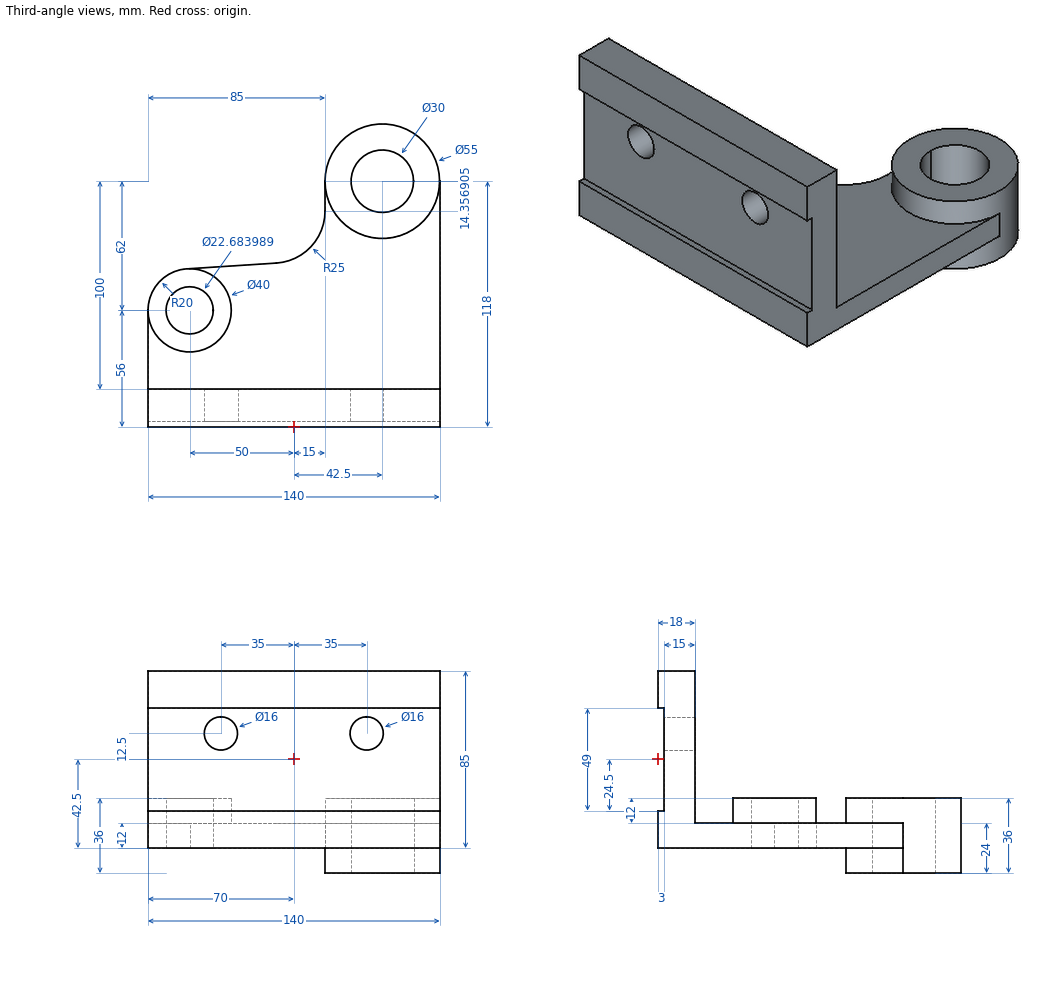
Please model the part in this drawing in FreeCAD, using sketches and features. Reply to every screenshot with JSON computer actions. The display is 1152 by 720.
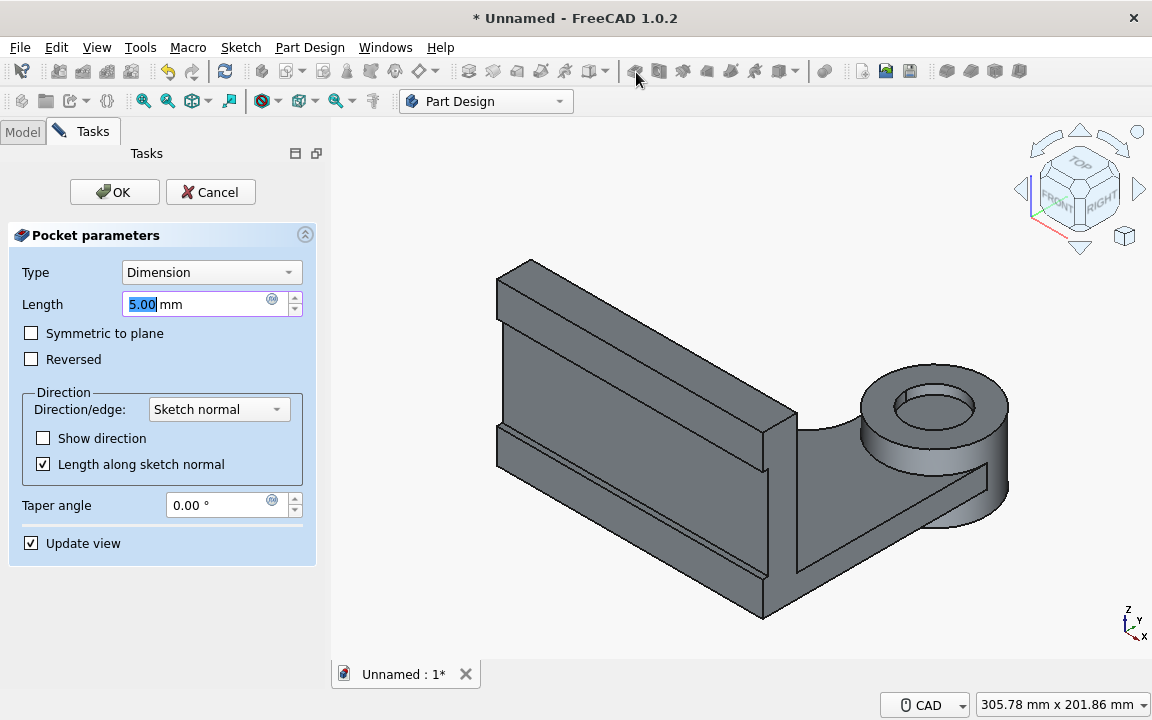
{"action": "type", "text": "36"}
{"action": "key", "text": "Tab"}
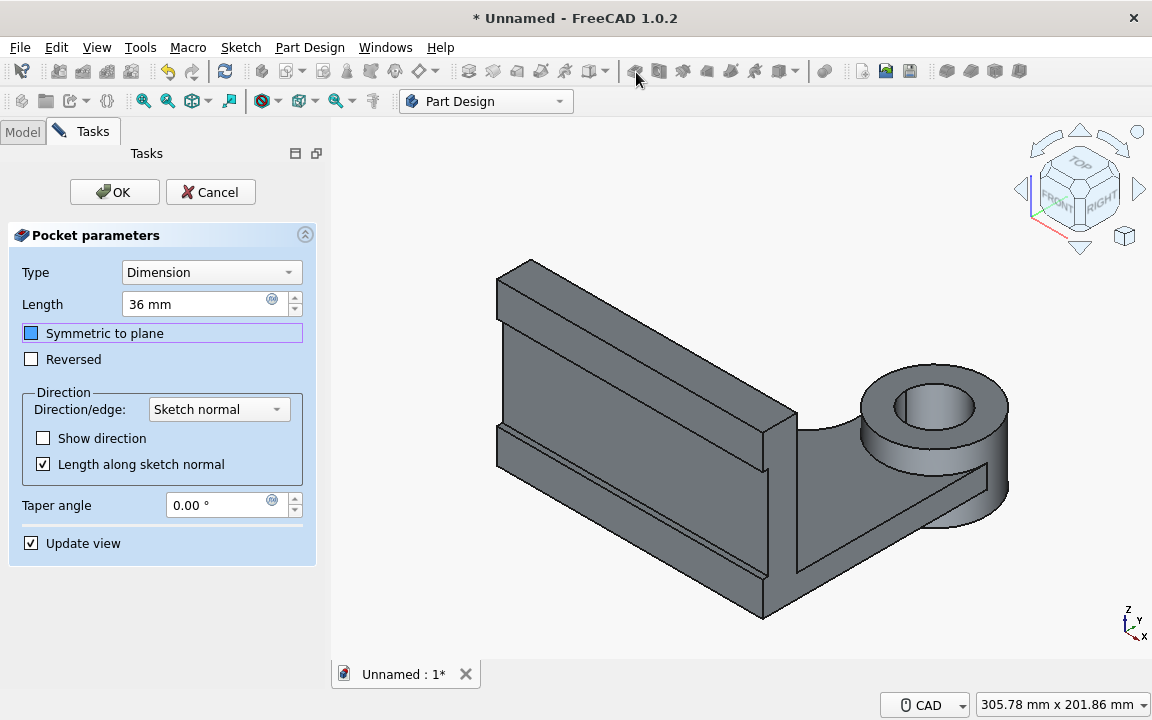
{"action": "left_click", "coordinate": [115, 192]}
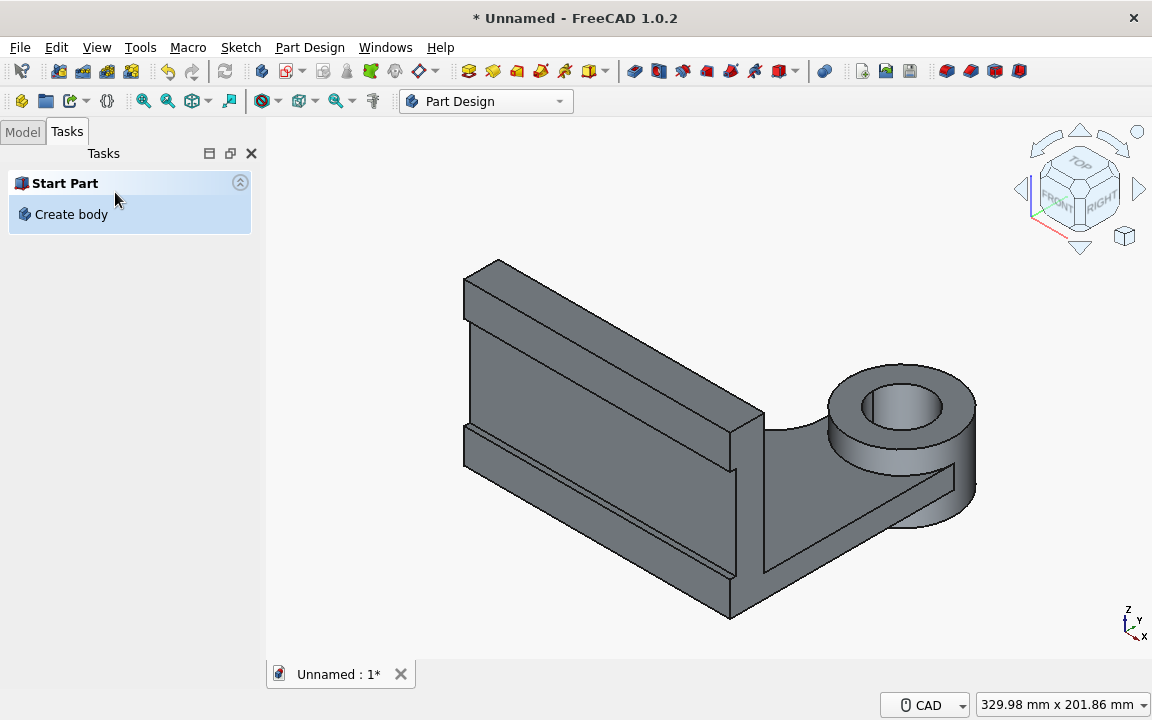
{"action": "left_click", "coordinate": [962, 406]}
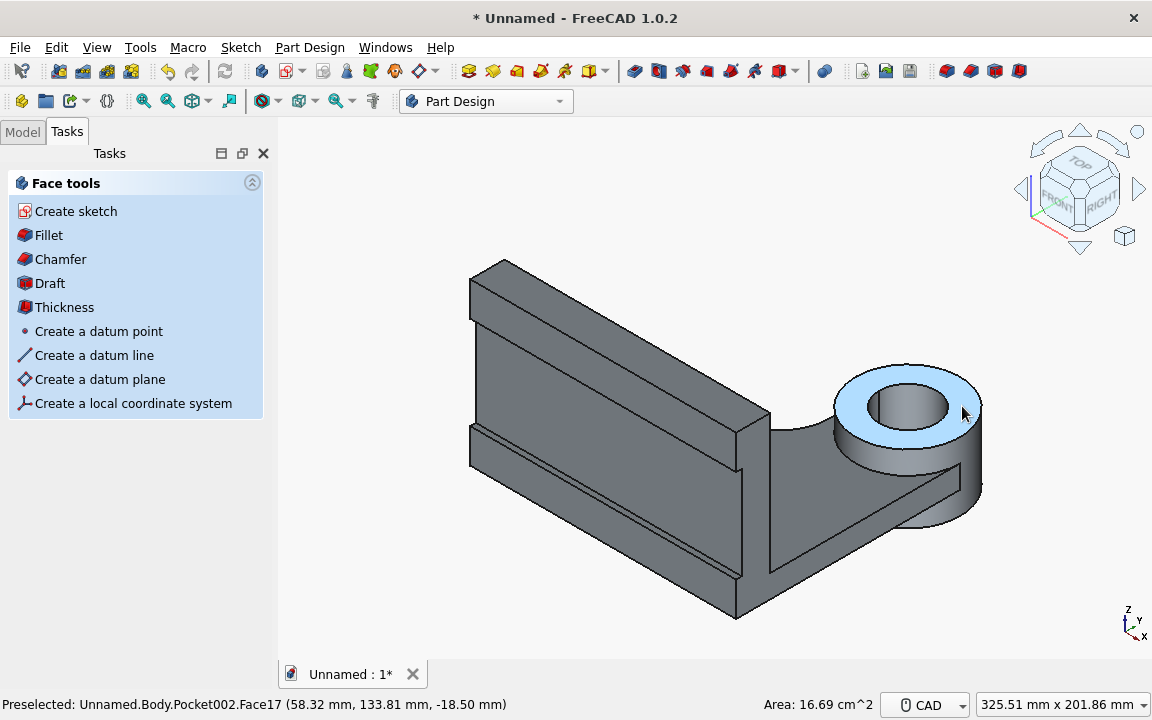
{"action": "left_click", "coordinate": [286, 72]}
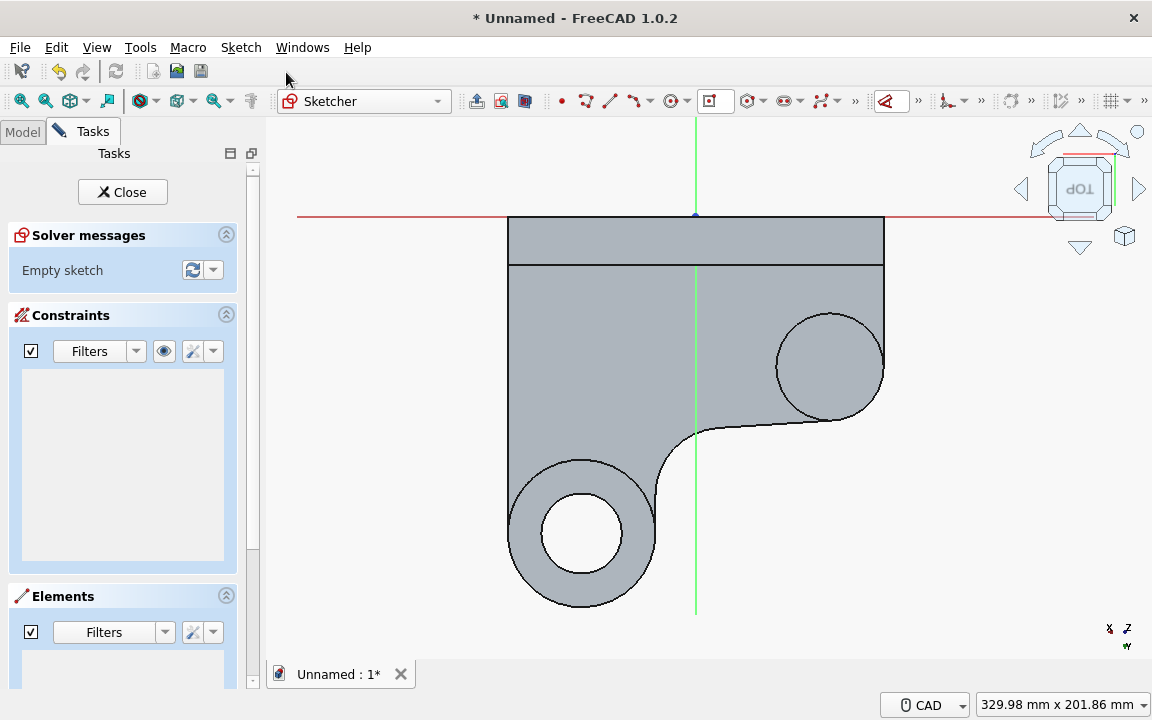
{"action": "scroll", "coordinate": [868, 363], "scroll_direction": "up", "scroll_amount": 9}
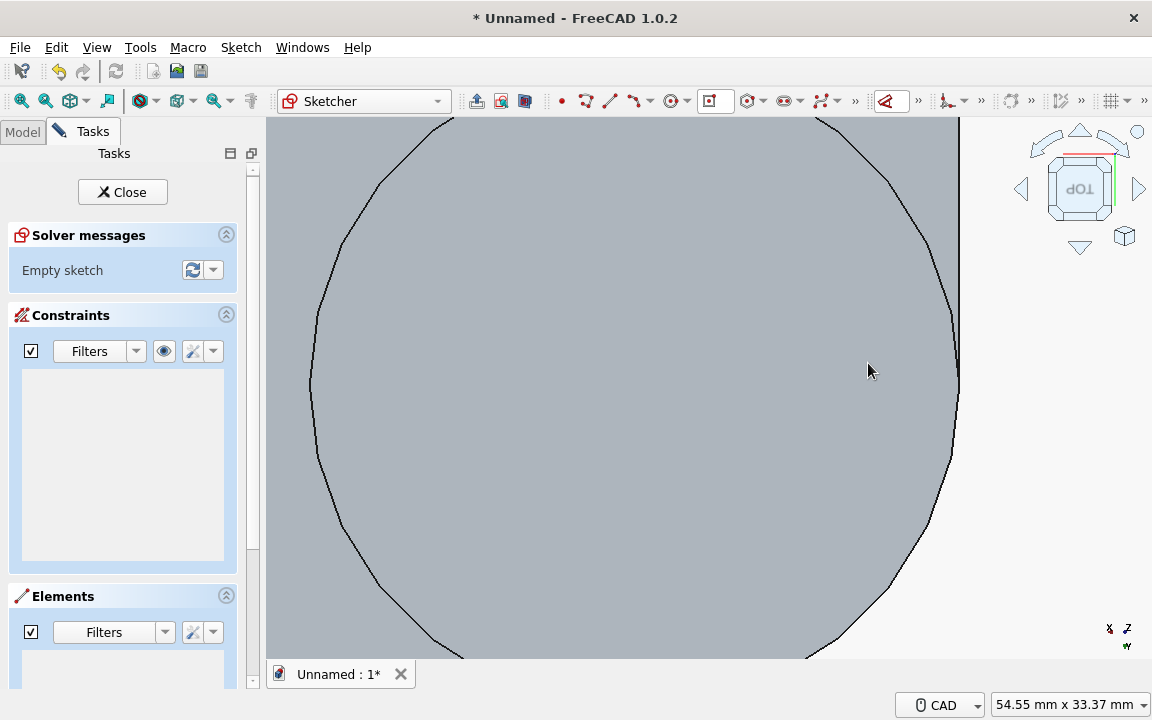
{"action": "left_click", "coordinate": [672, 102]}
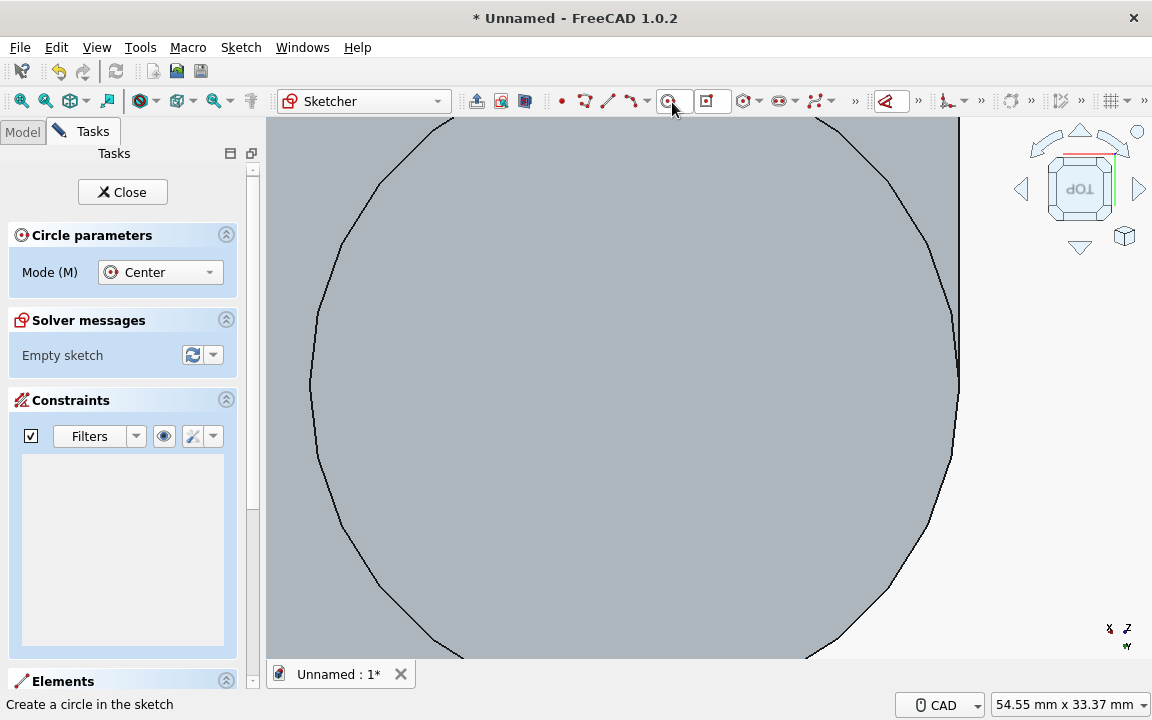
{"action": "left_click", "coordinate": [635, 385]}
{"action": "left_click", "coordinate": [765, 255]}
{"action": "key", "text": "Escape"}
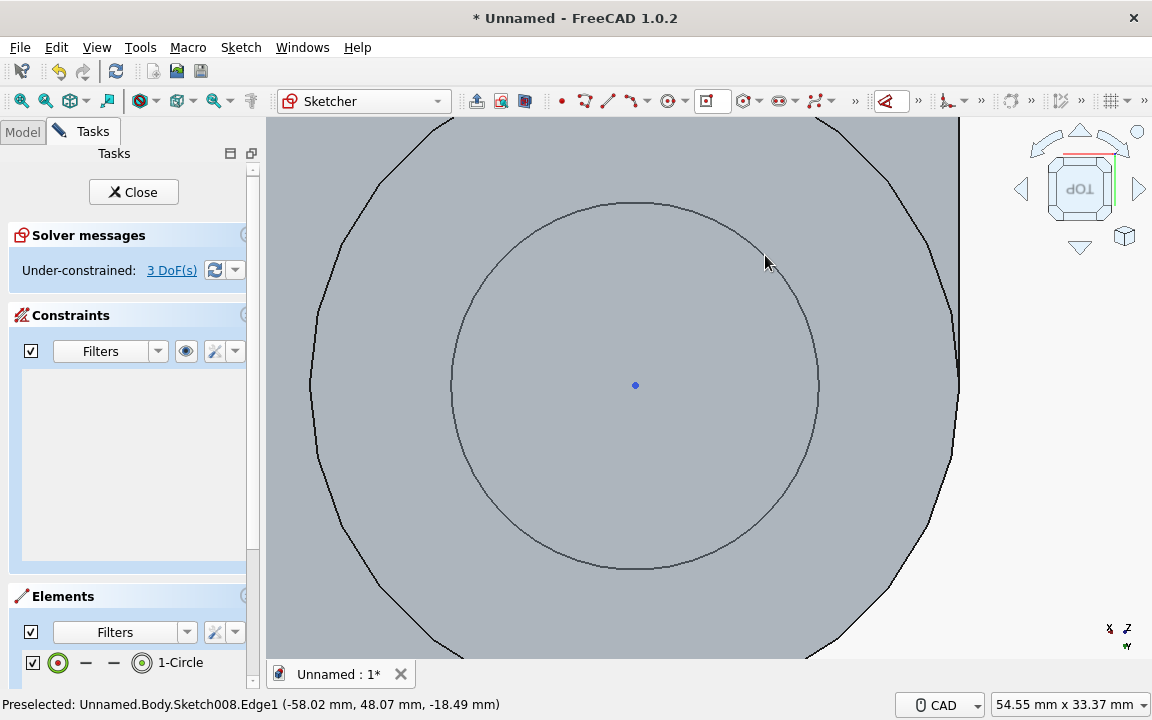
{"action": "left_click", "coordinate": [765, 256]}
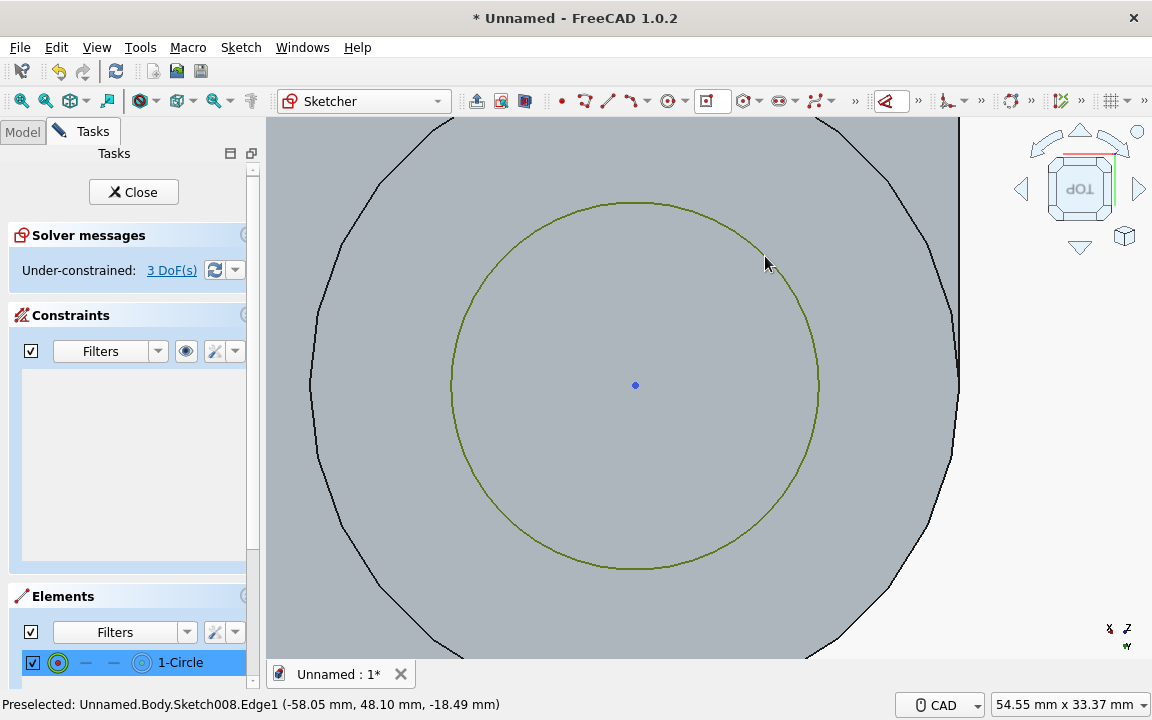
{"action": "key", "text": "k o"}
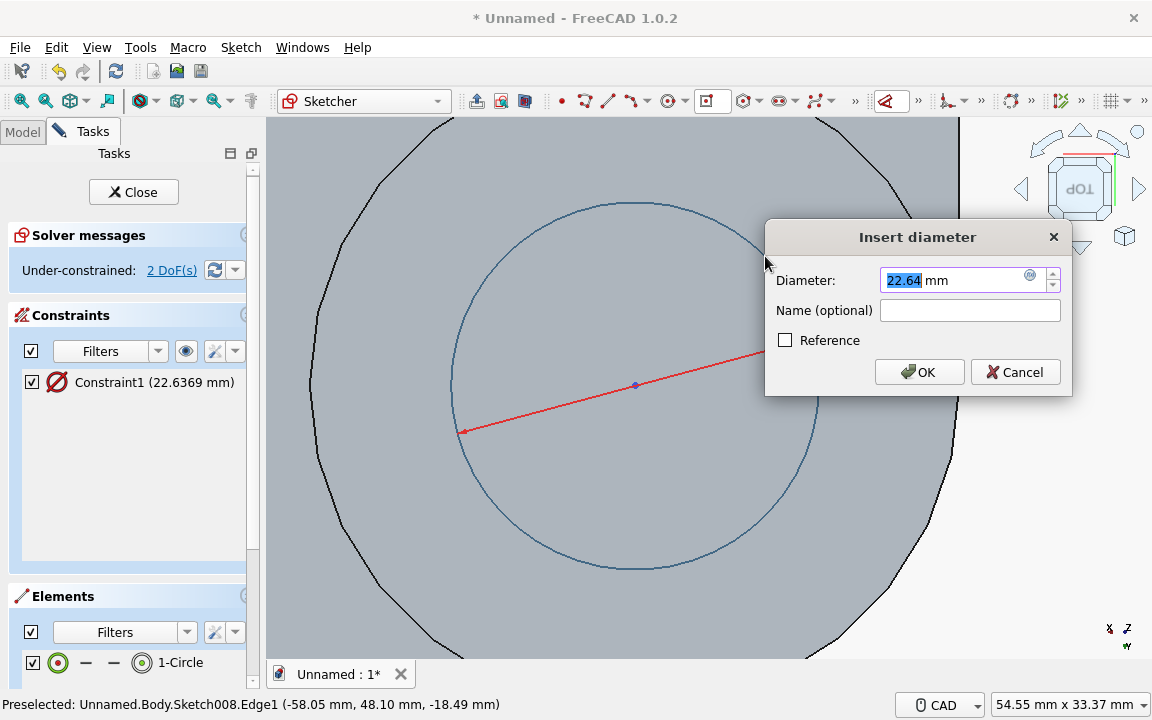
{"action": "type", "text": "22.683989"}
{"action": "key", "text": "Return"}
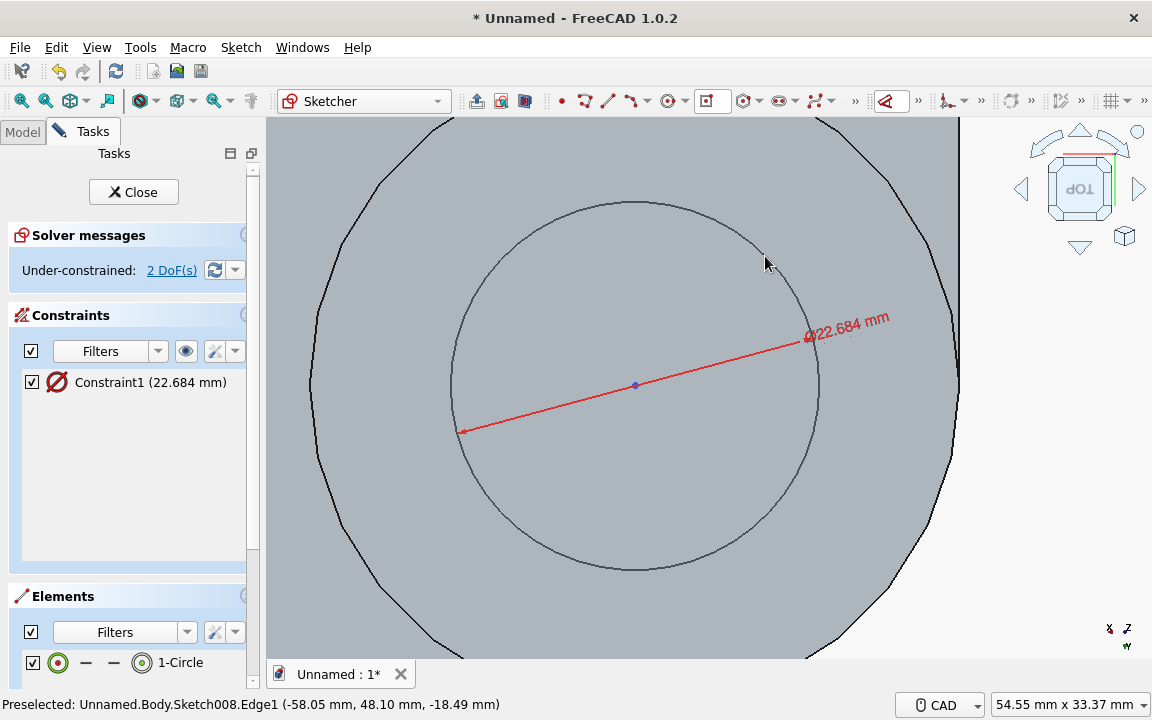
{"action": "left_click", "coordinate": [635, 386]}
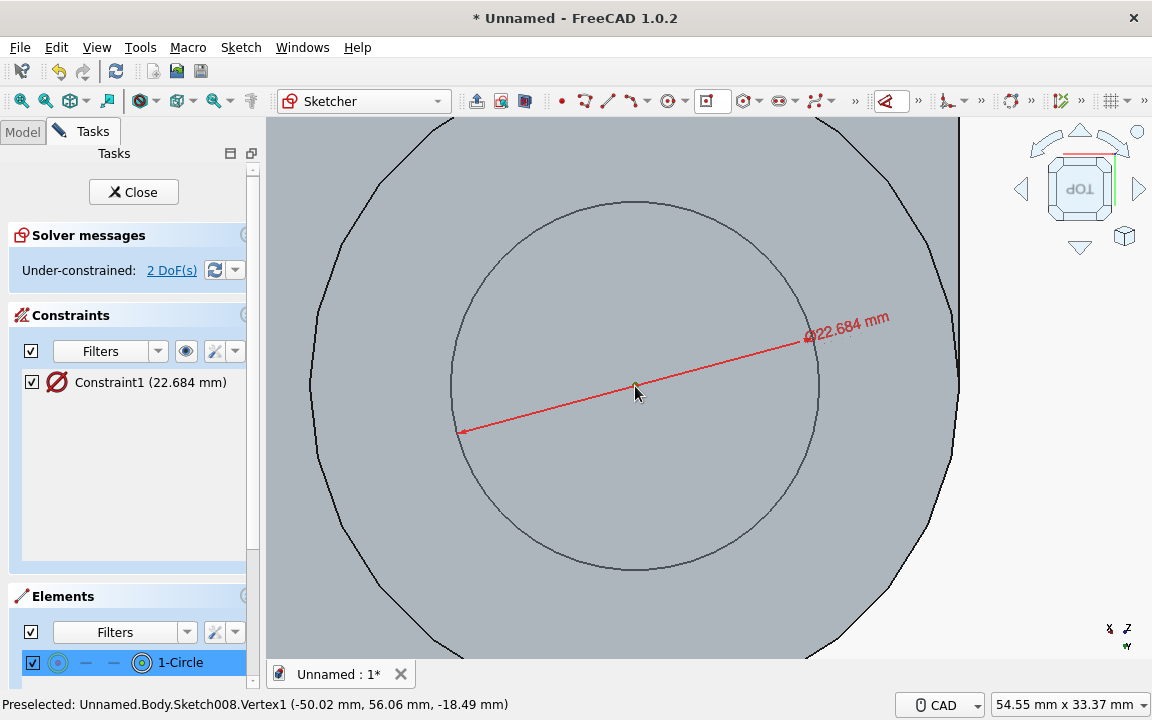
{"action": "key", "text": "l"}